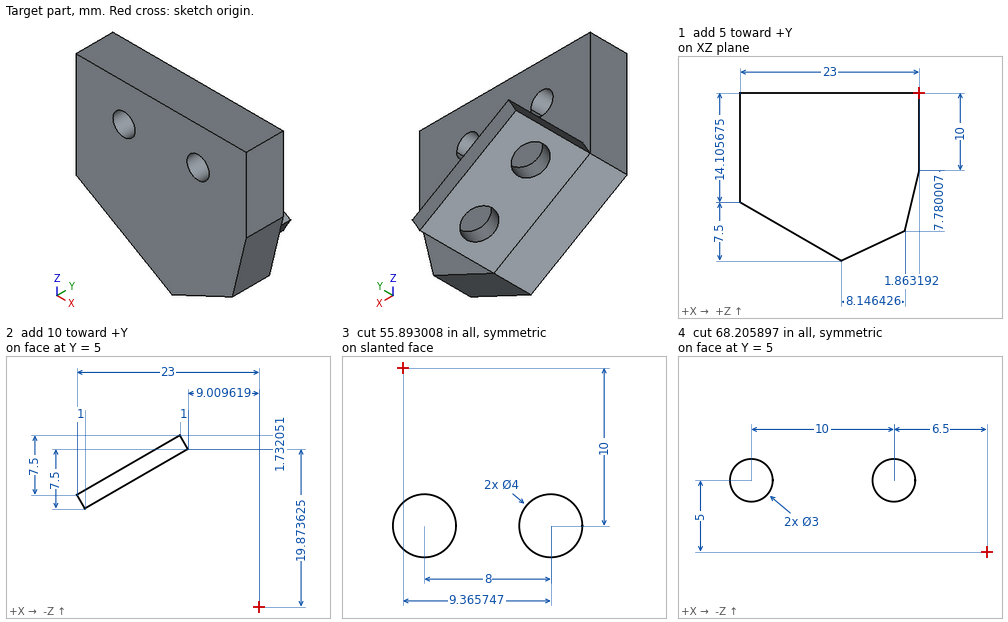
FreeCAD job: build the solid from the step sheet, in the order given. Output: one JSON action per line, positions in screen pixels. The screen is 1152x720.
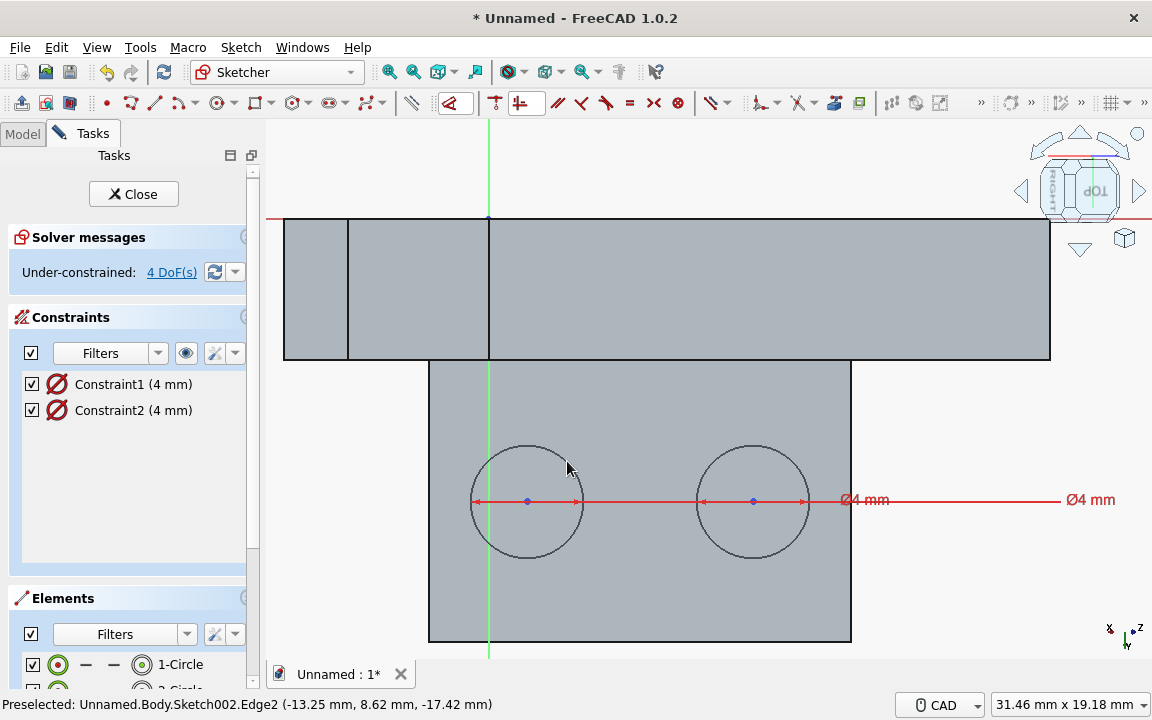
{"action": "left_click", "coordinate": [753, 502]}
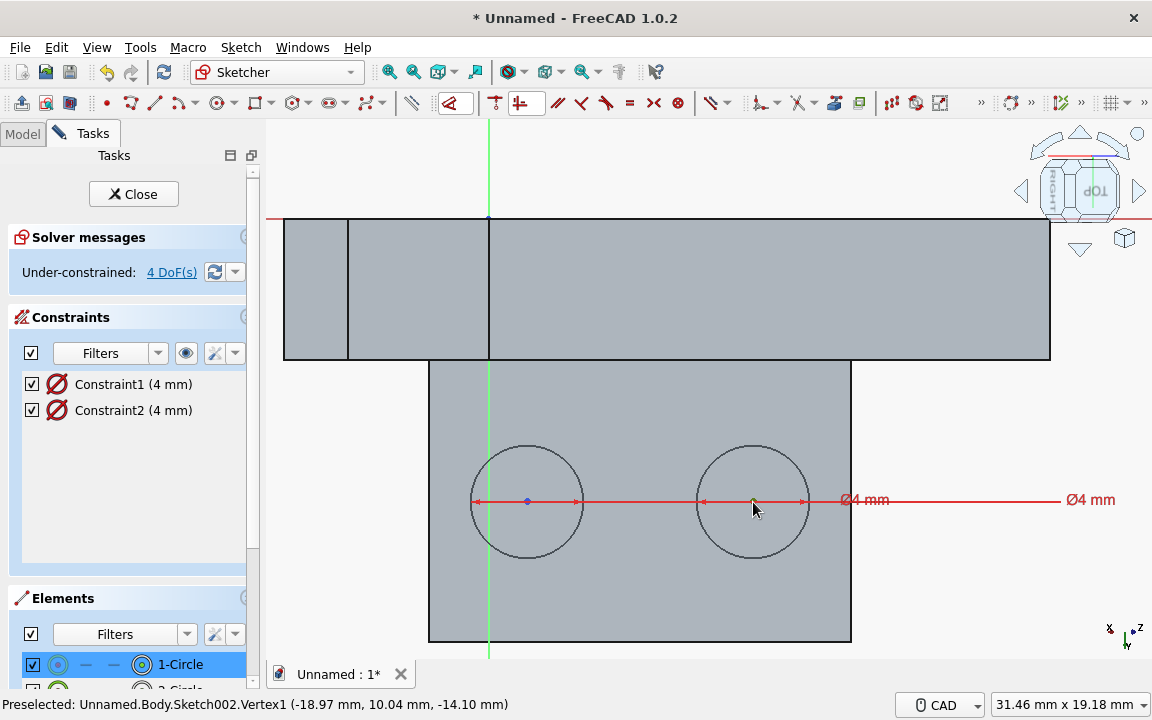
{"action": "left_click", "coordinate": [527, 502]}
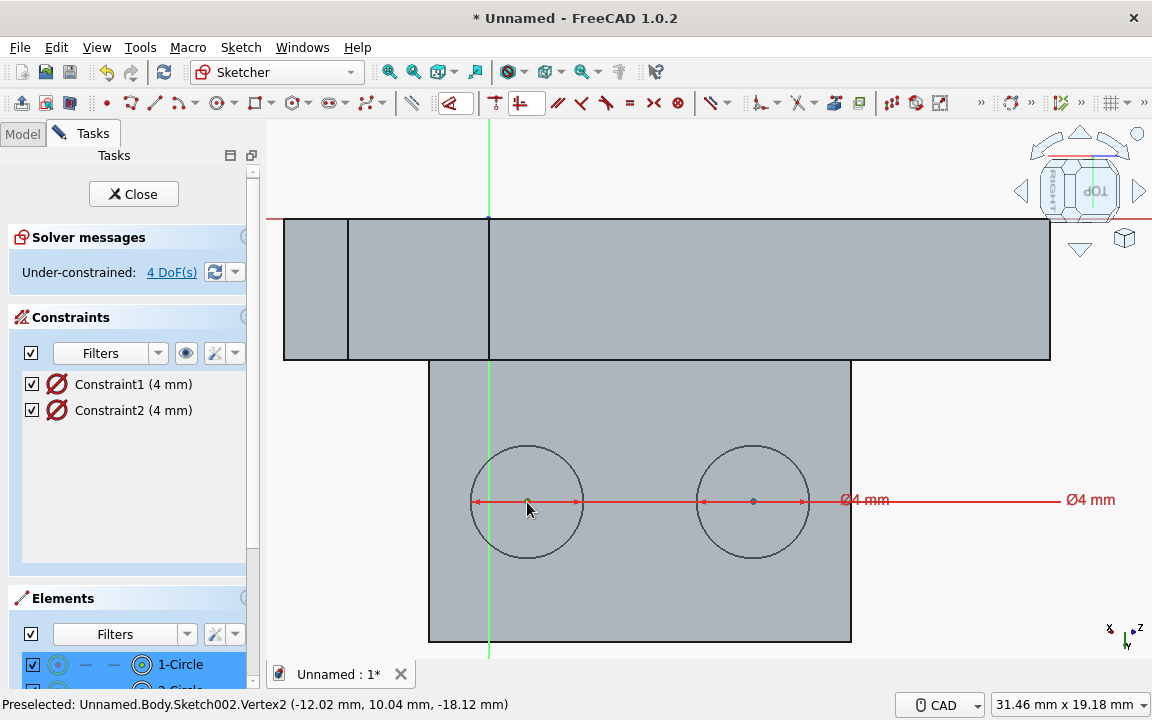
{"action": "key", "text": "h"}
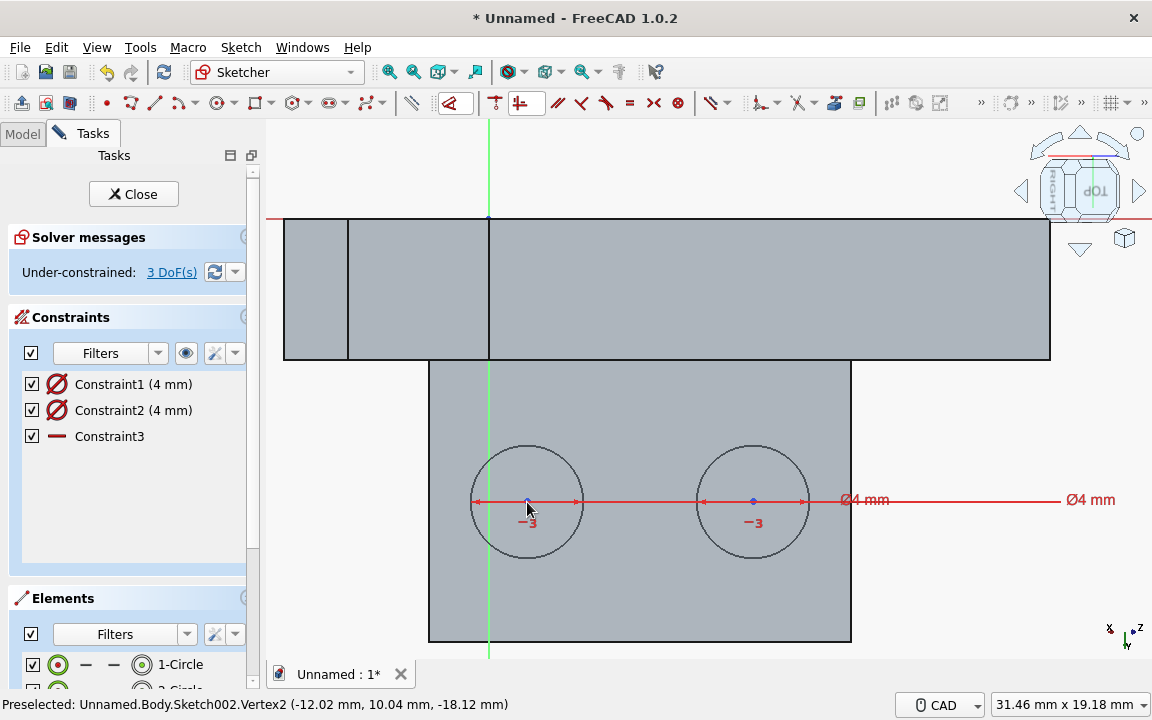
{"action": "left_click", "coordinate": [753, 502]}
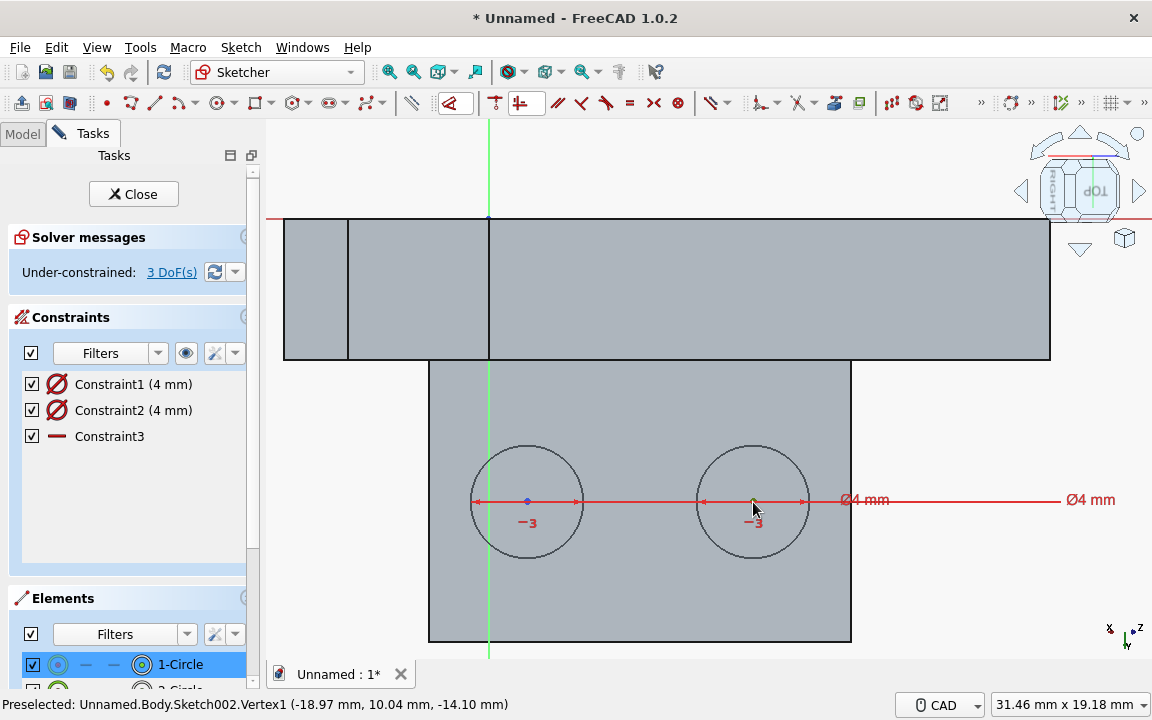
{"action": "left_click", "coordinate": [468, 104]}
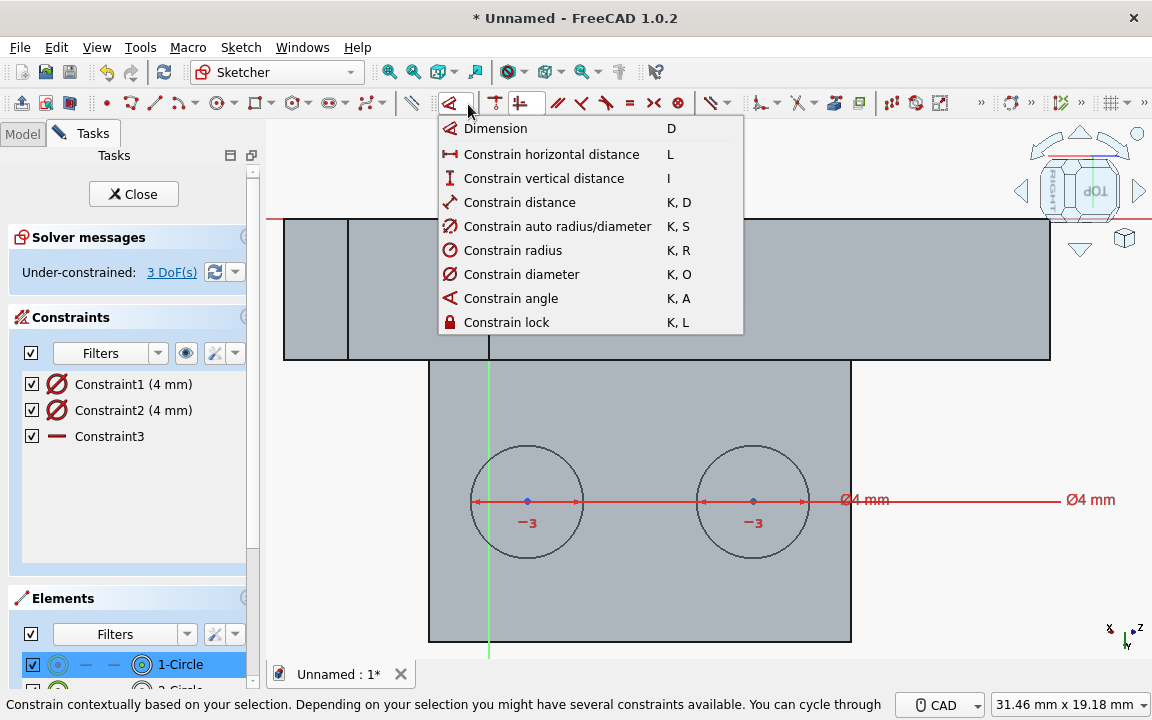
{"action": "left_click", "coordinate": [591, 178]}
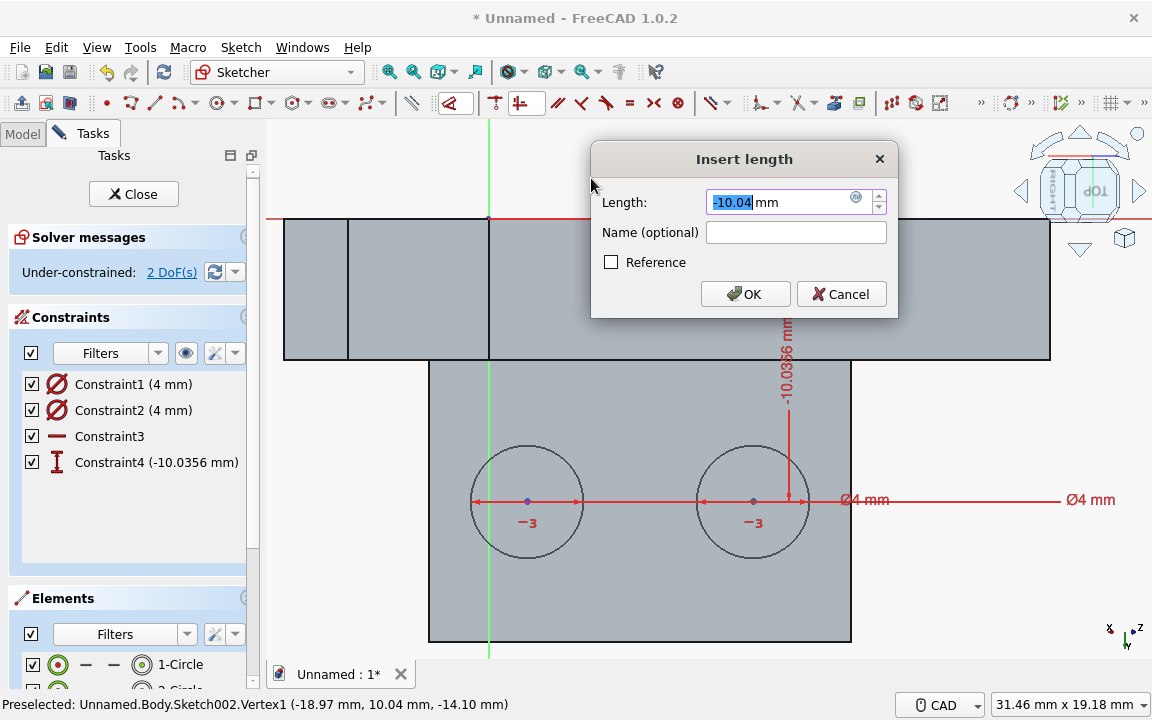
{"action": "type", "text": "-10"}
{"action": "key", "text": "Return"}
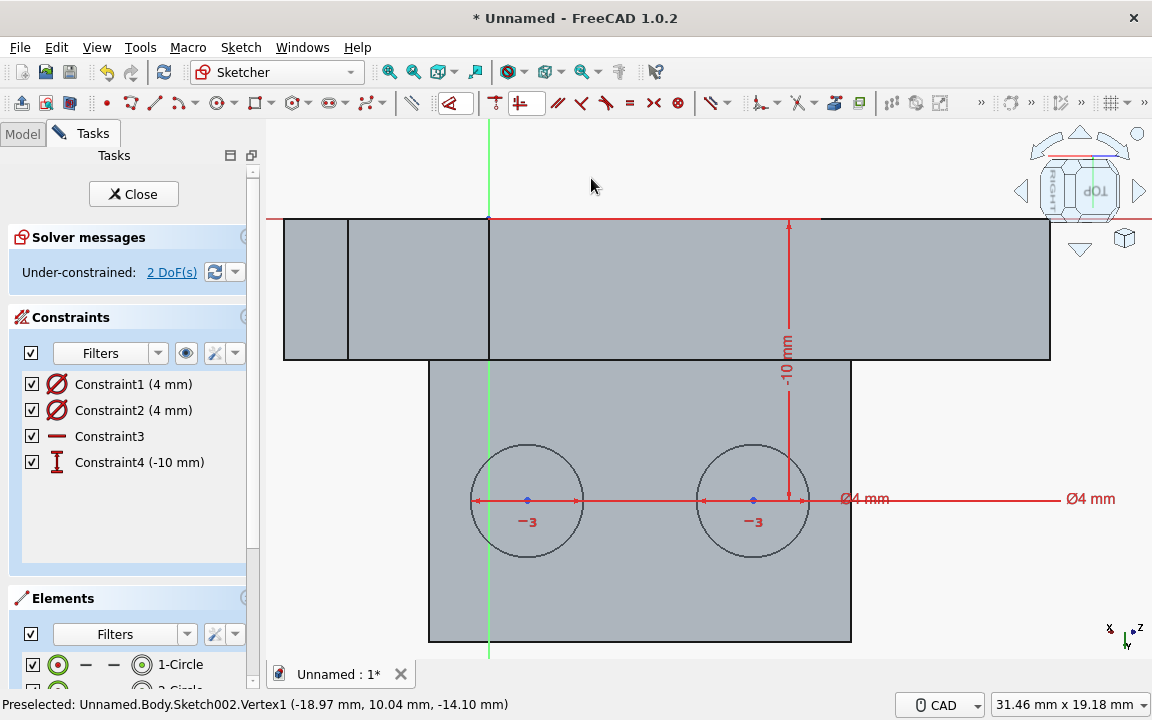
{"action": "left_click", "coordinate": [753, 501]}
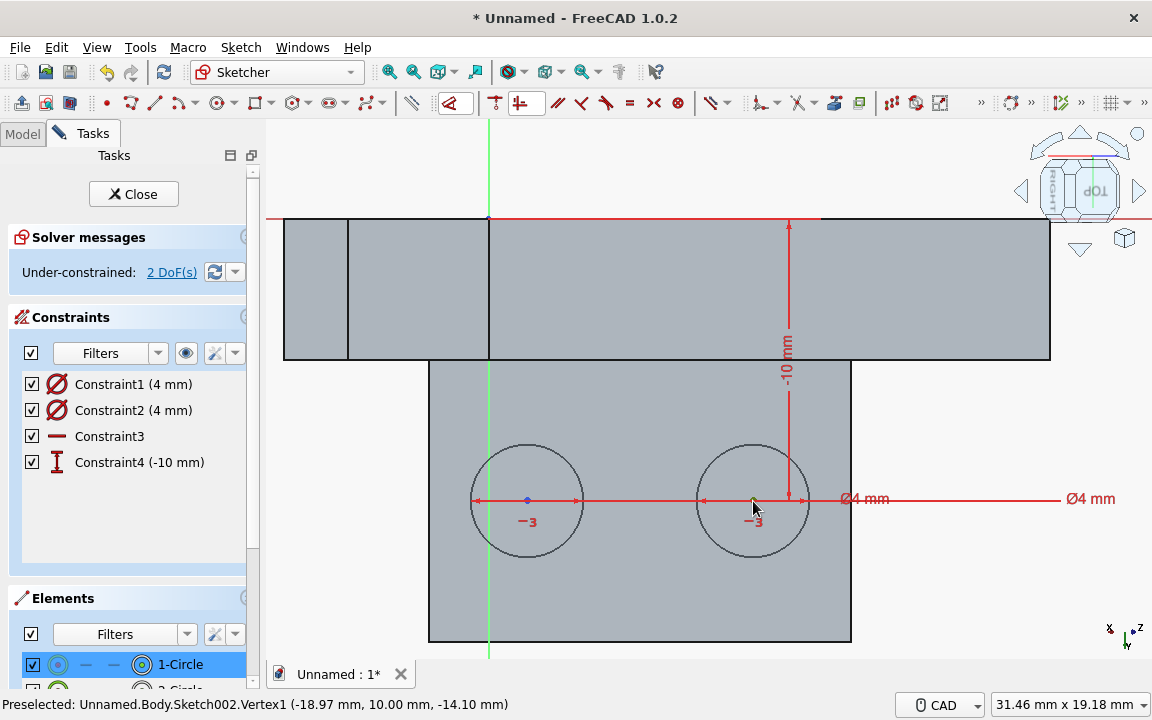
{"action": "left_click", "coordinate": [527, 501]}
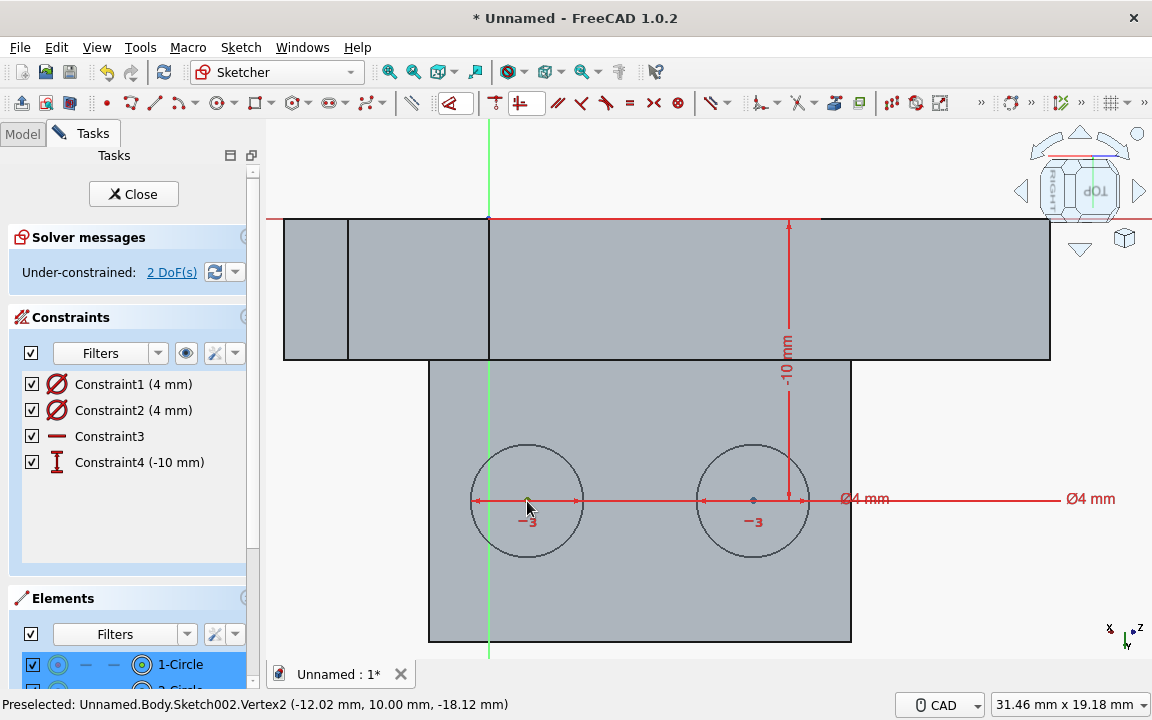
{"action": "left_click", "coordinate": [468, 104]}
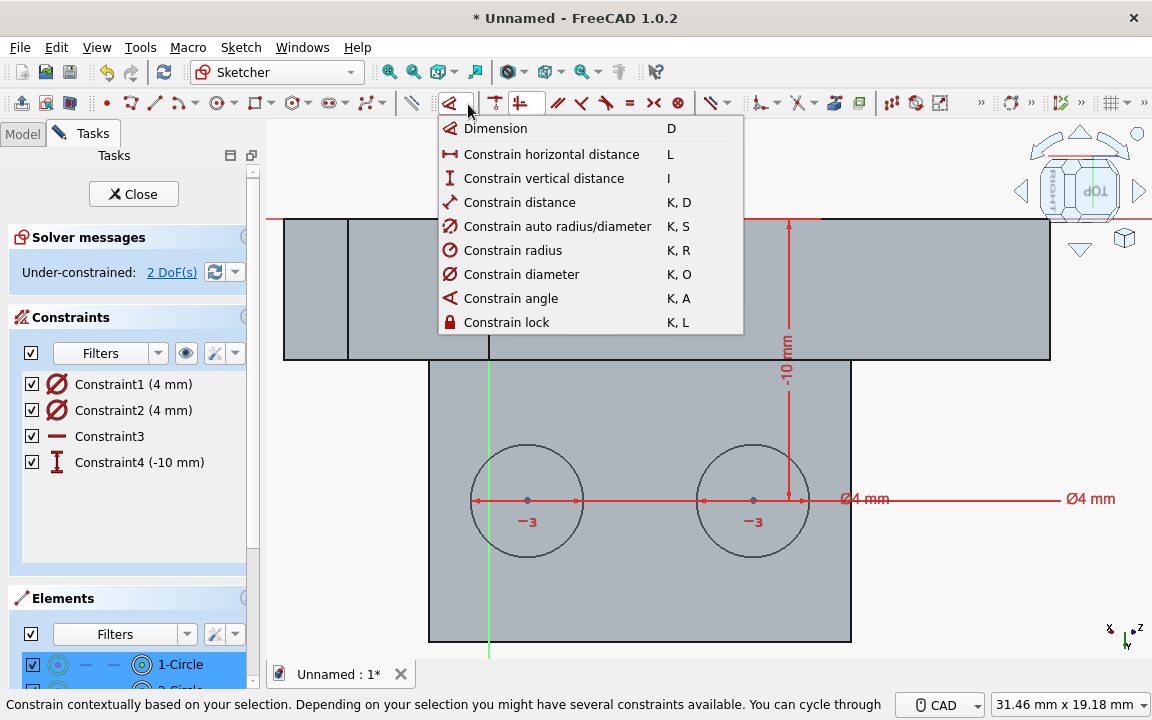
{"action": "left_click", "coordinate": [591, 154]}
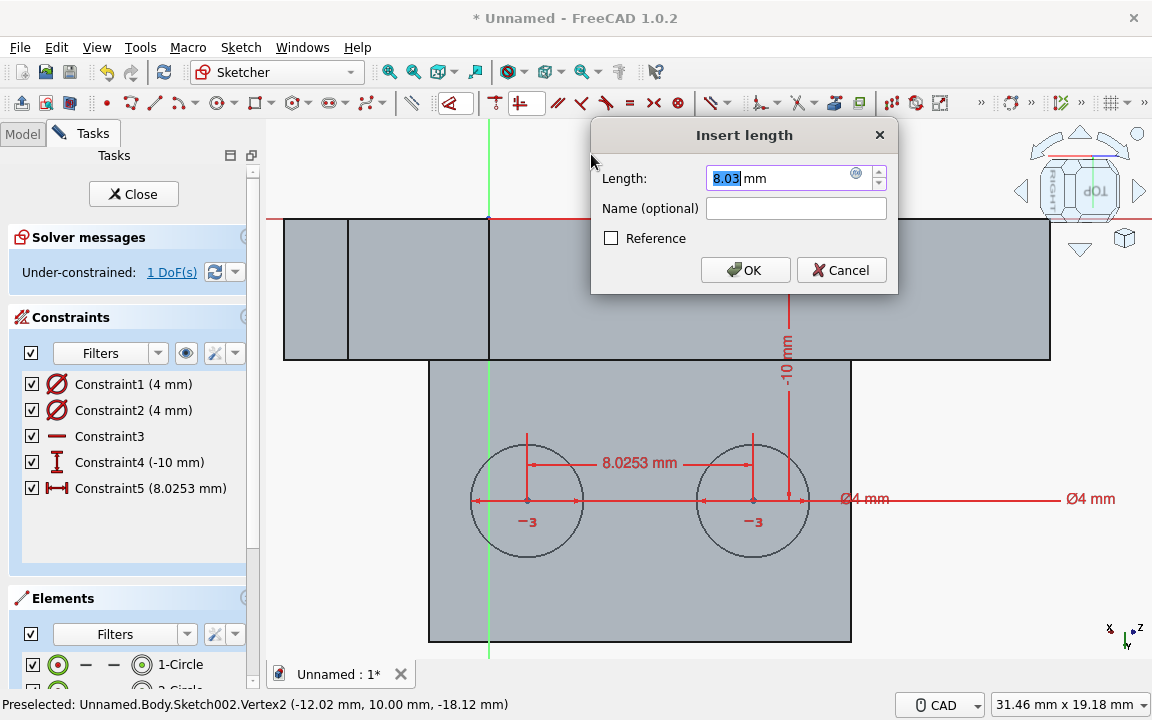
{"action": "type", "text": "8"}
{"action": "key", "text": "Return"}